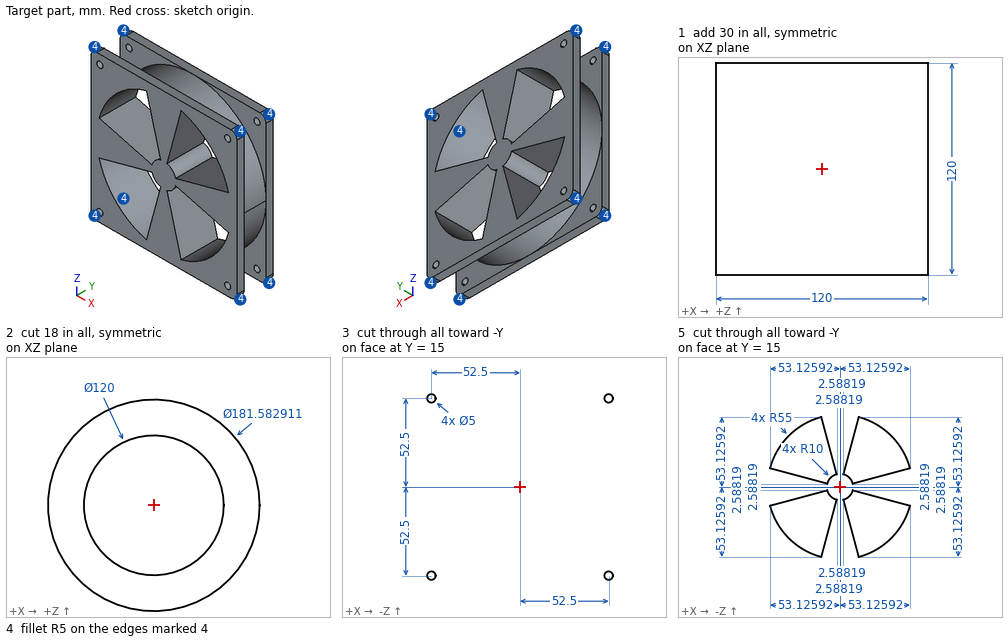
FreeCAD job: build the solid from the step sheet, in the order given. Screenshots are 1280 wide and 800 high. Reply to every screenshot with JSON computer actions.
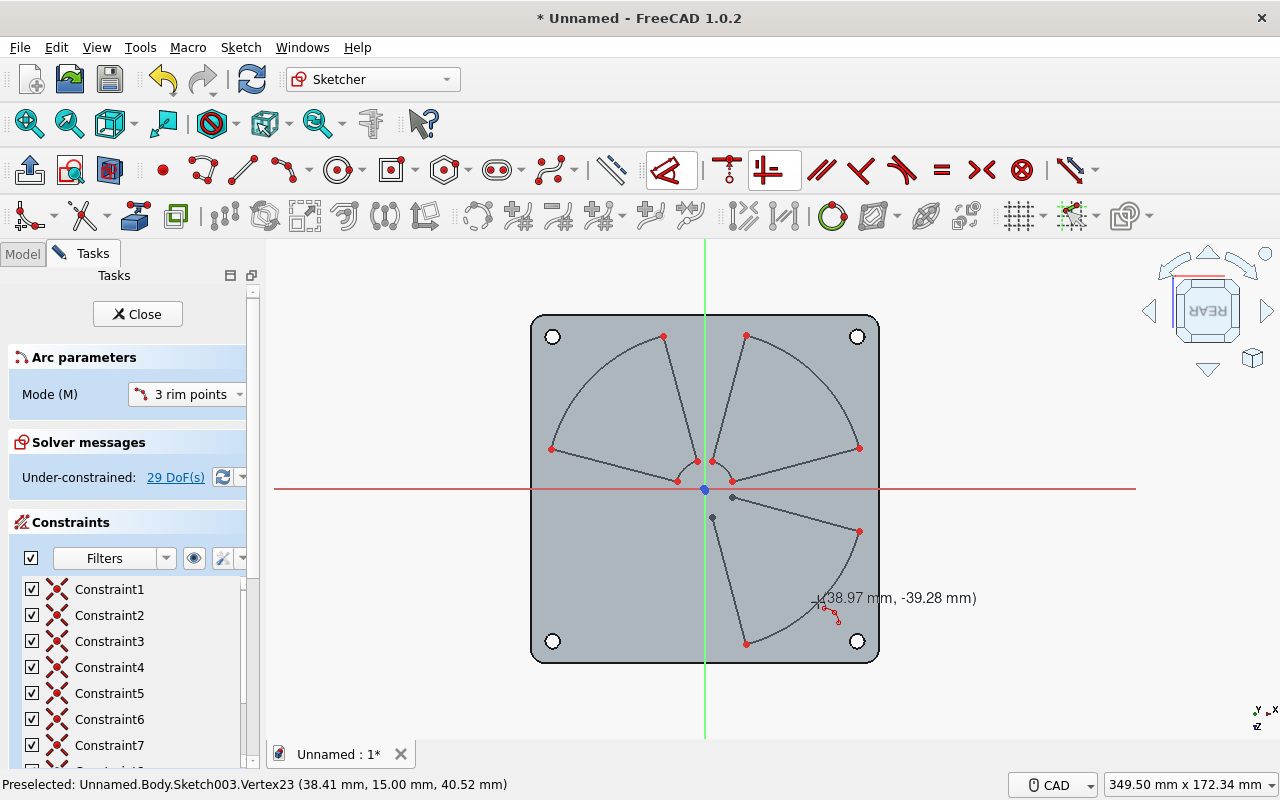
{"action": "scroll", "coordinate": [733, 497], "scroll_direction": "up", "scroll_amount": 4}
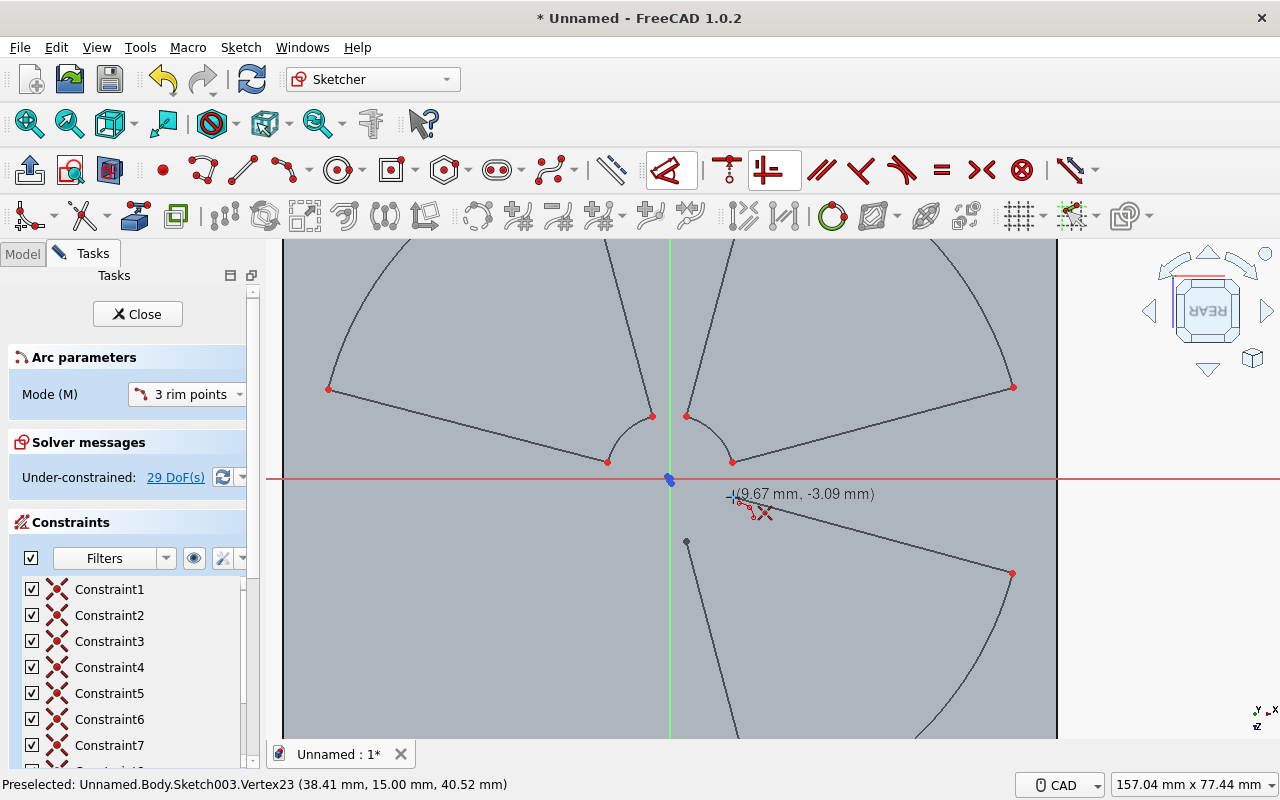
{"action": "left_click", "coordinate": [732, 497]}
{"action": "left_click", "coordinate": [686, 542]}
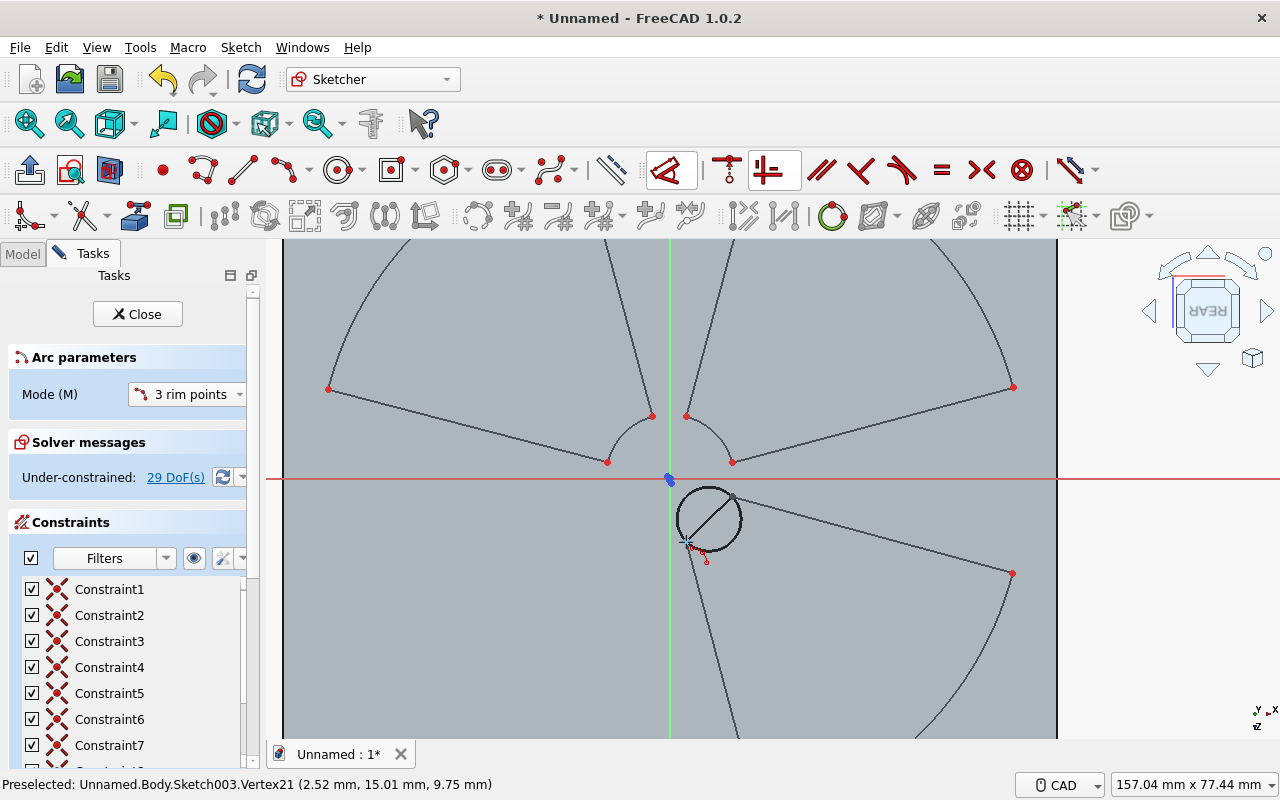
{"action": "scroll", "coordinate": [716, 524], "scroll_direction": "up", "scroll_amount": 4}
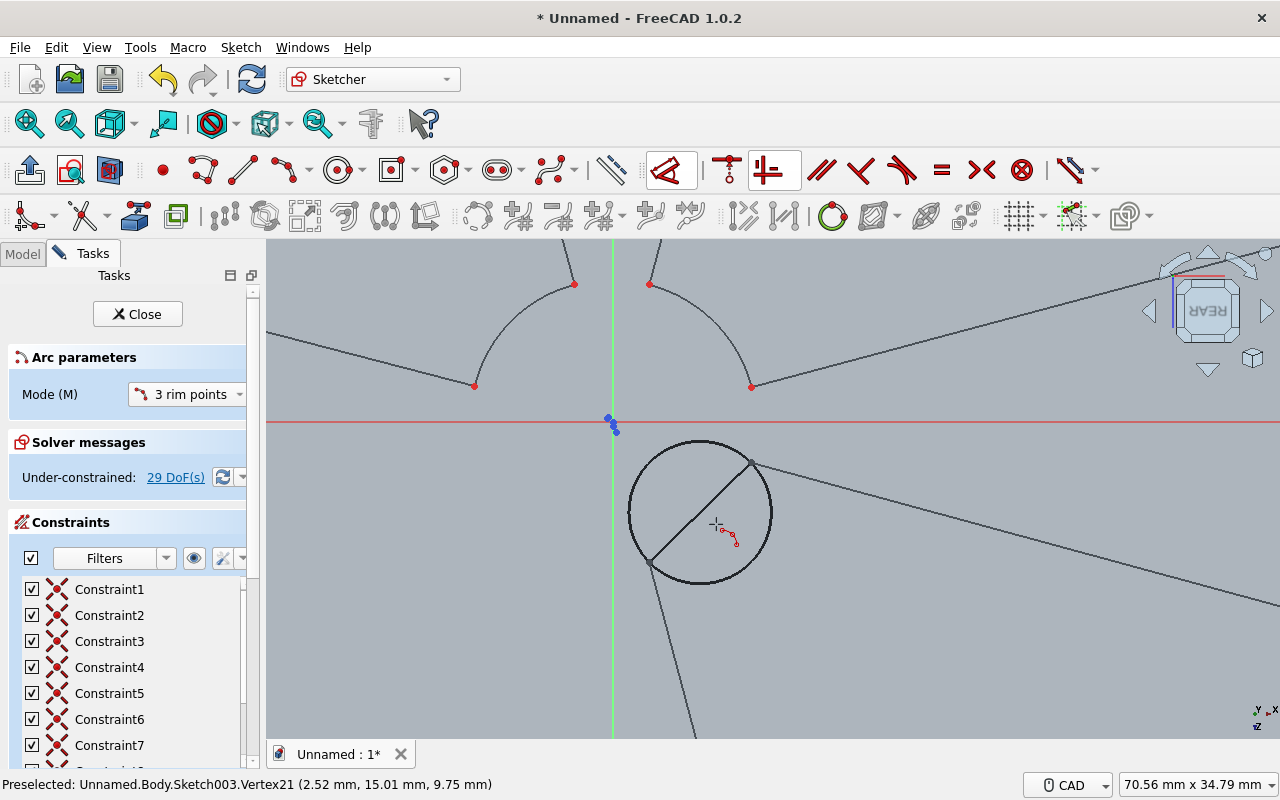
{"action": "left_click", "coordinate": [715, 524]}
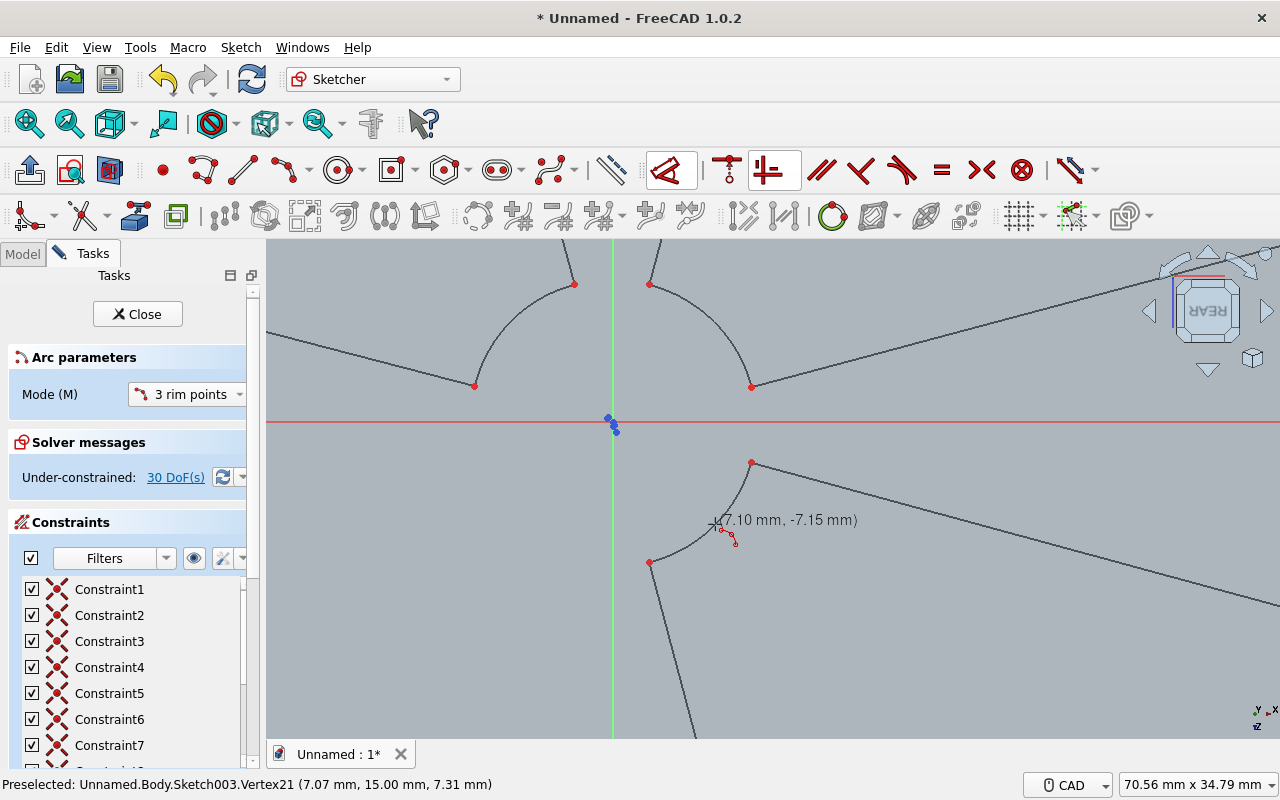
{"action": "left_click", "coordinate": [244, 170]}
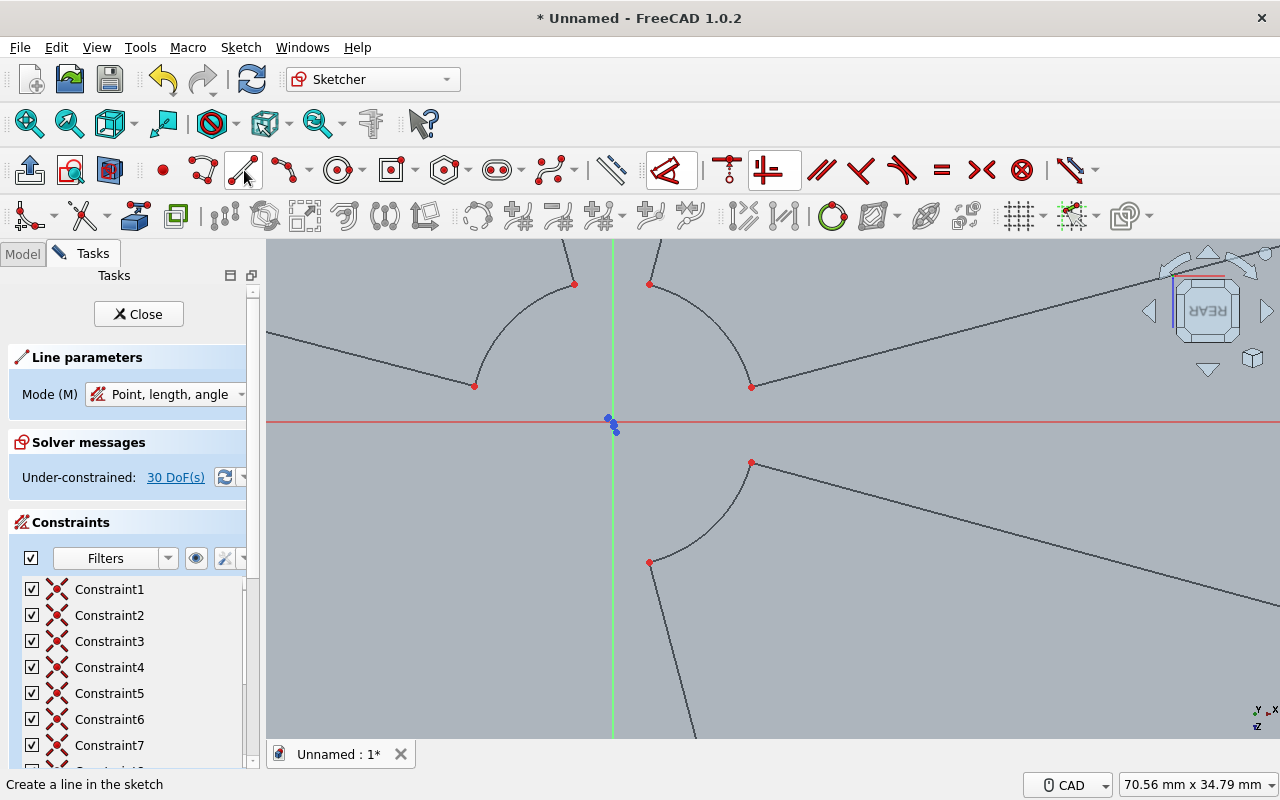
{"action": "scroll", "coordinate": [728, 506], "scroll_direction": "down", "scroll_amount": 8}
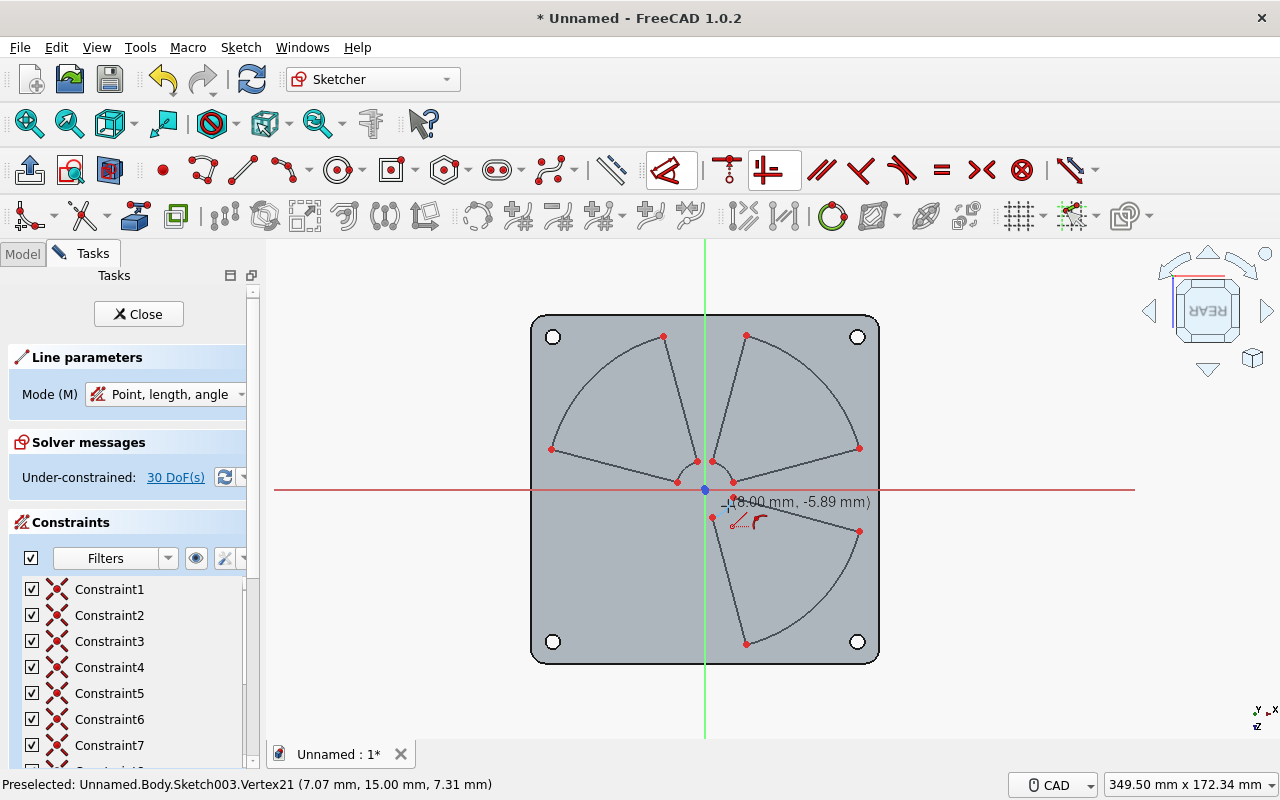
{"action": "left_click", "coordinate": [664, 644]}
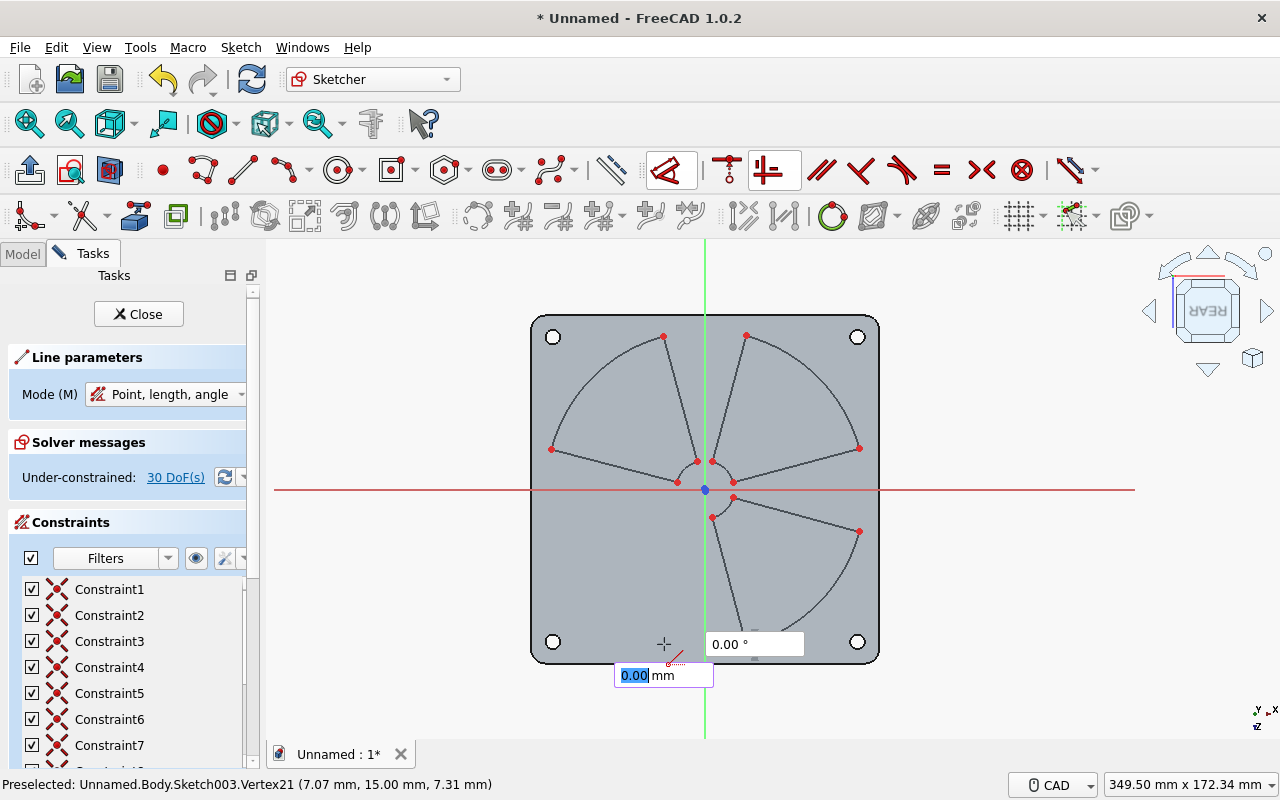
{"action": "scroll", "coordinate": [698, 518], "scroll_direction": "up", "scroll_amount": 4}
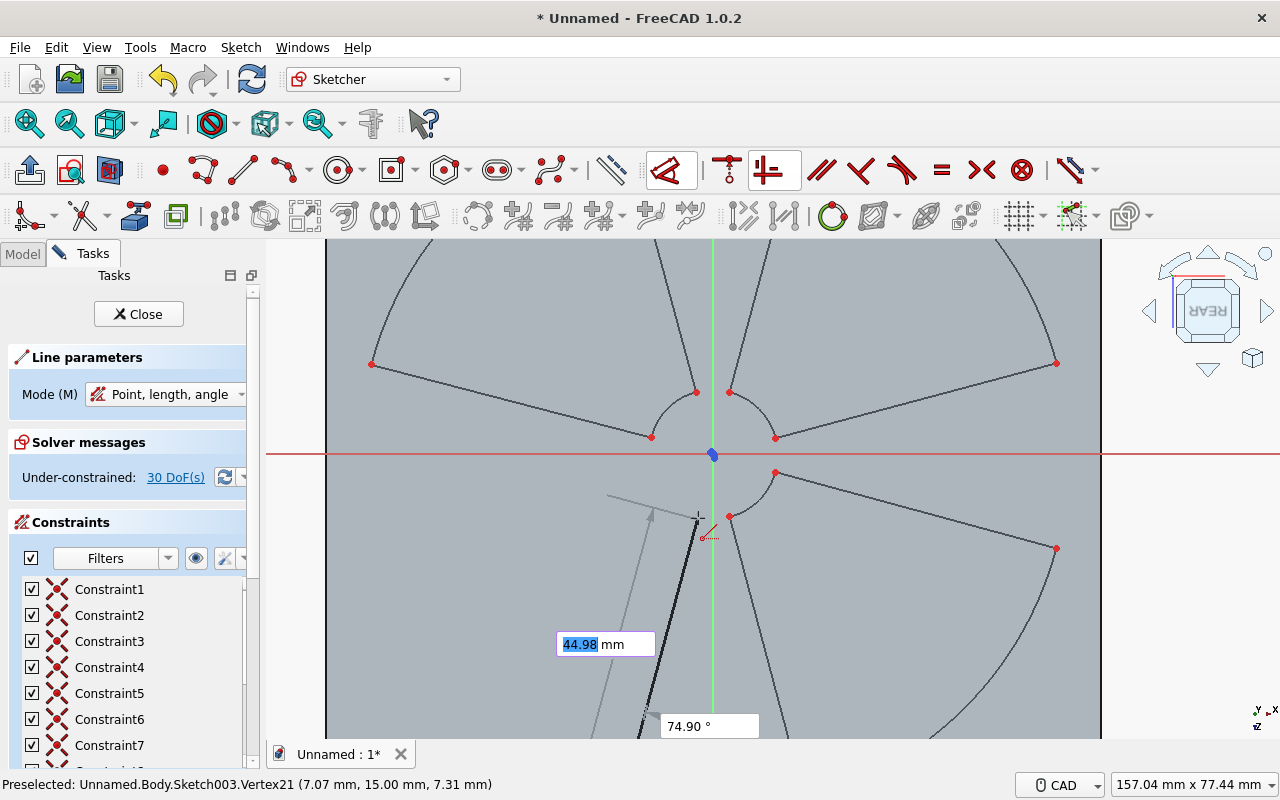
{"action": "left_click", "coordinate": [697, 516]}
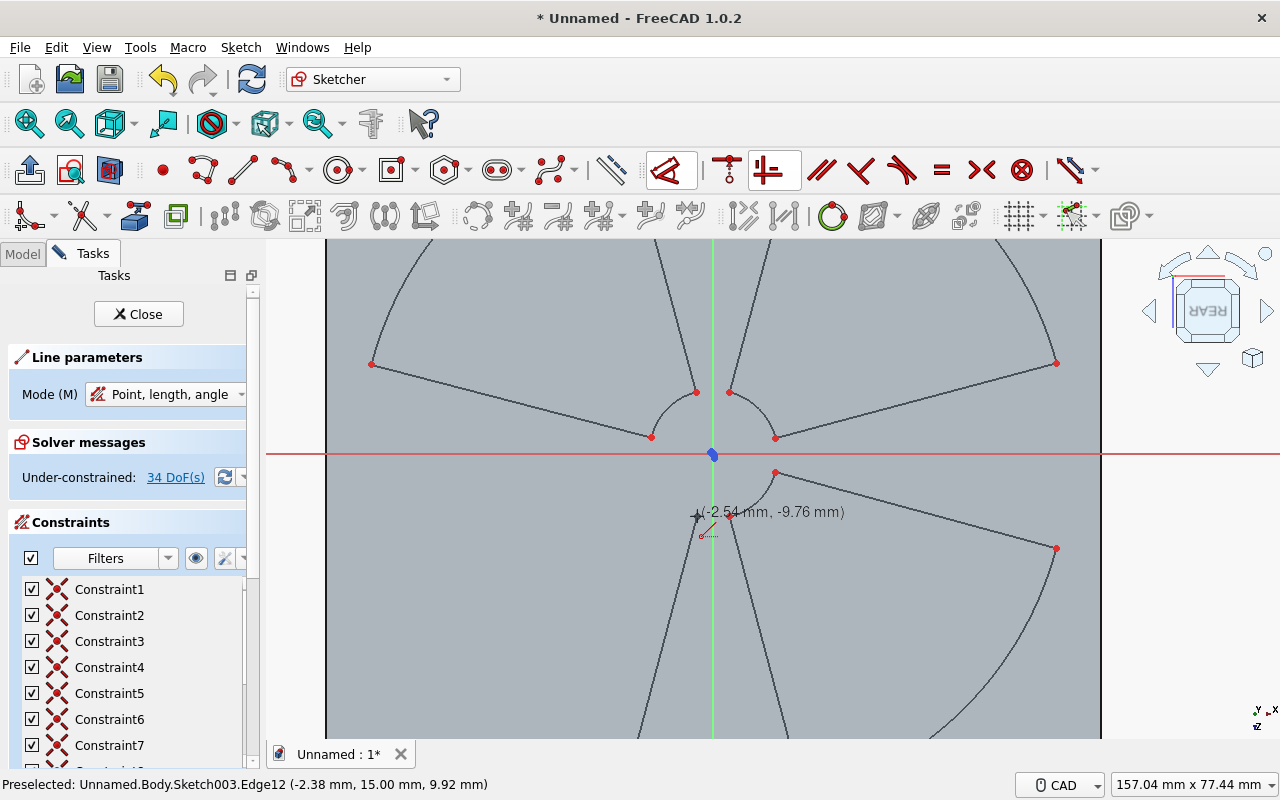
{"action": "left_click", "coordinate": [651, 471]}
{"action": "left_click", "coordinate": [370, 546]}